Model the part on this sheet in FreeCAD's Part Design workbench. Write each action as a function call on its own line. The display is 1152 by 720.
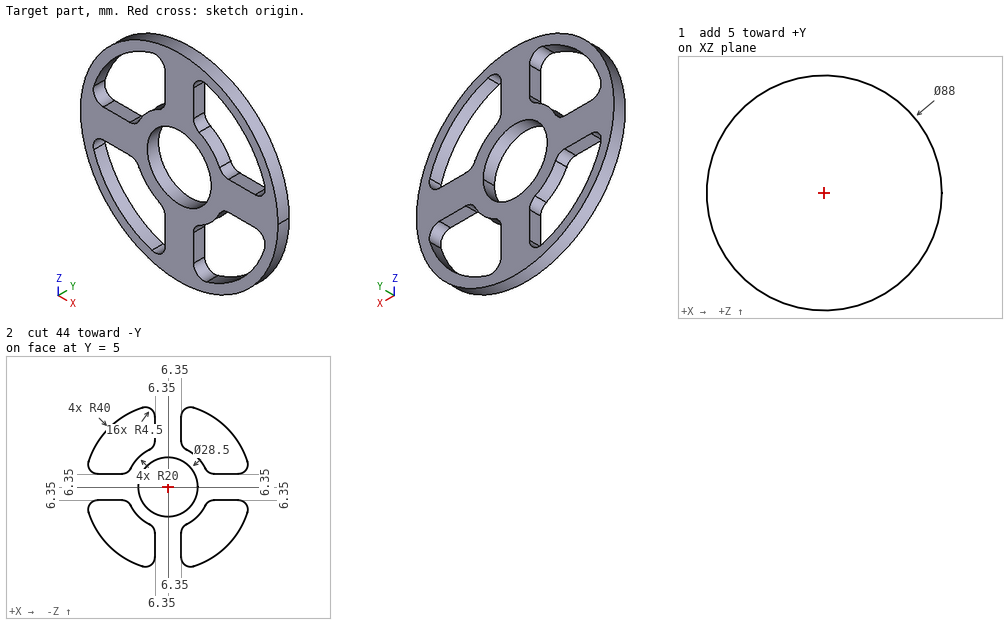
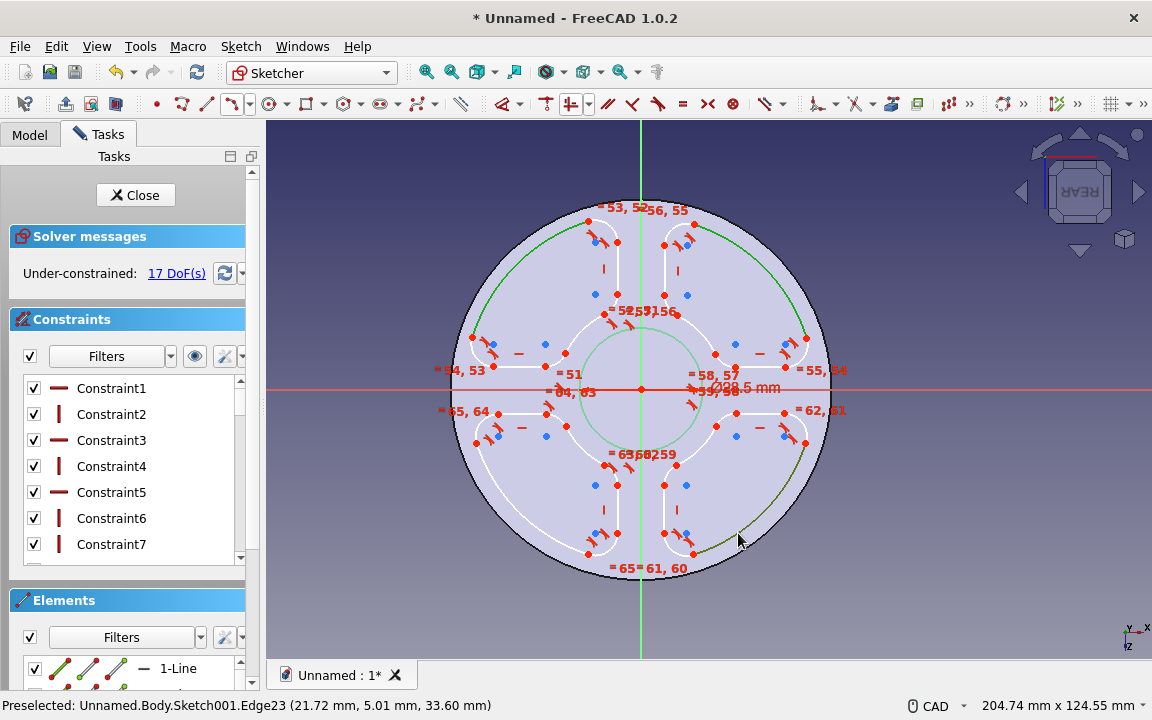
click(499, 488)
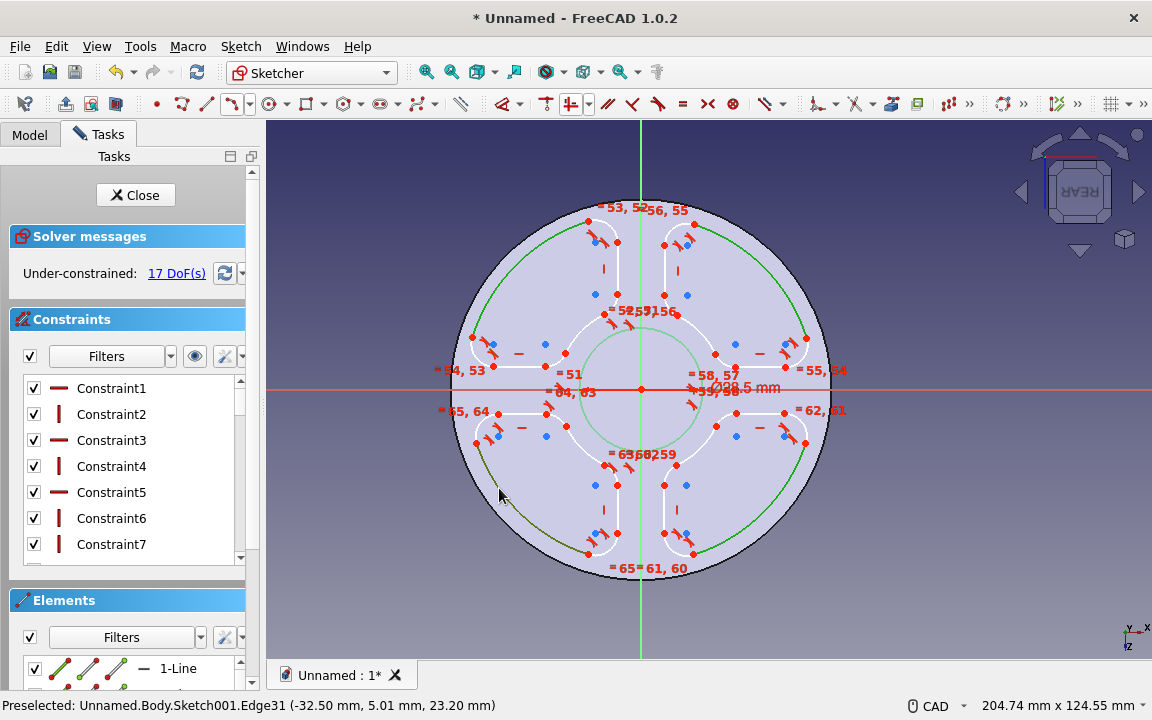
key(e)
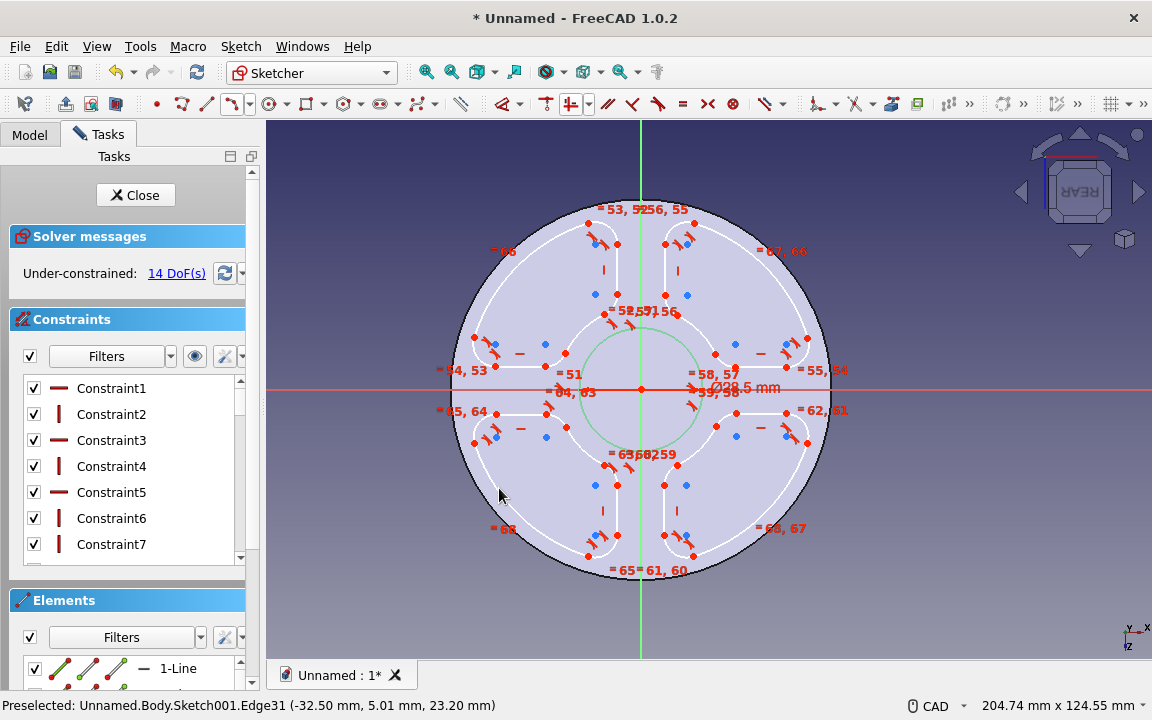
click(590, 323)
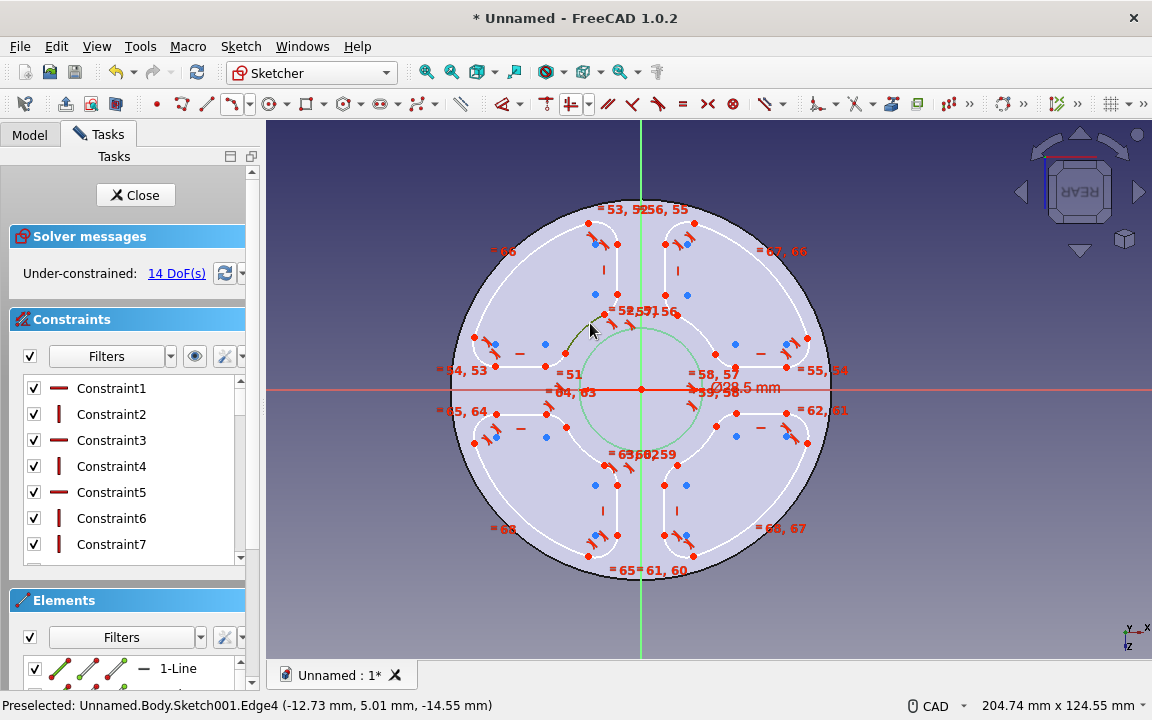
click(707, 340)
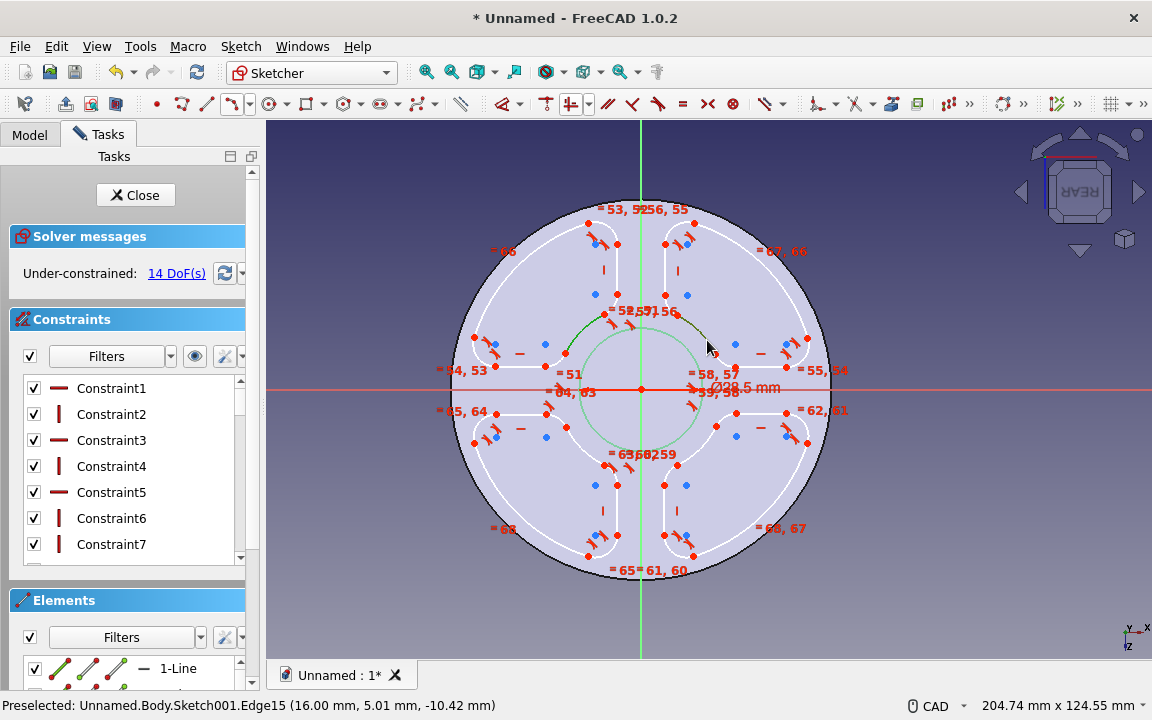
click(691, 457)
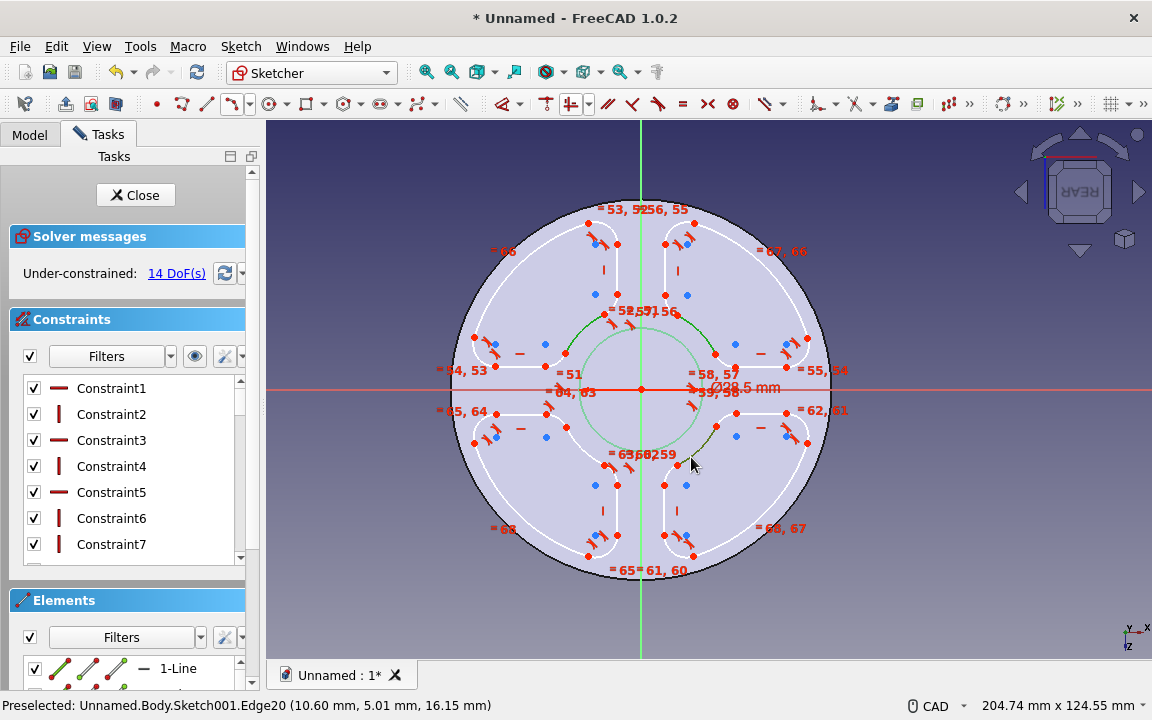
click(575, 441)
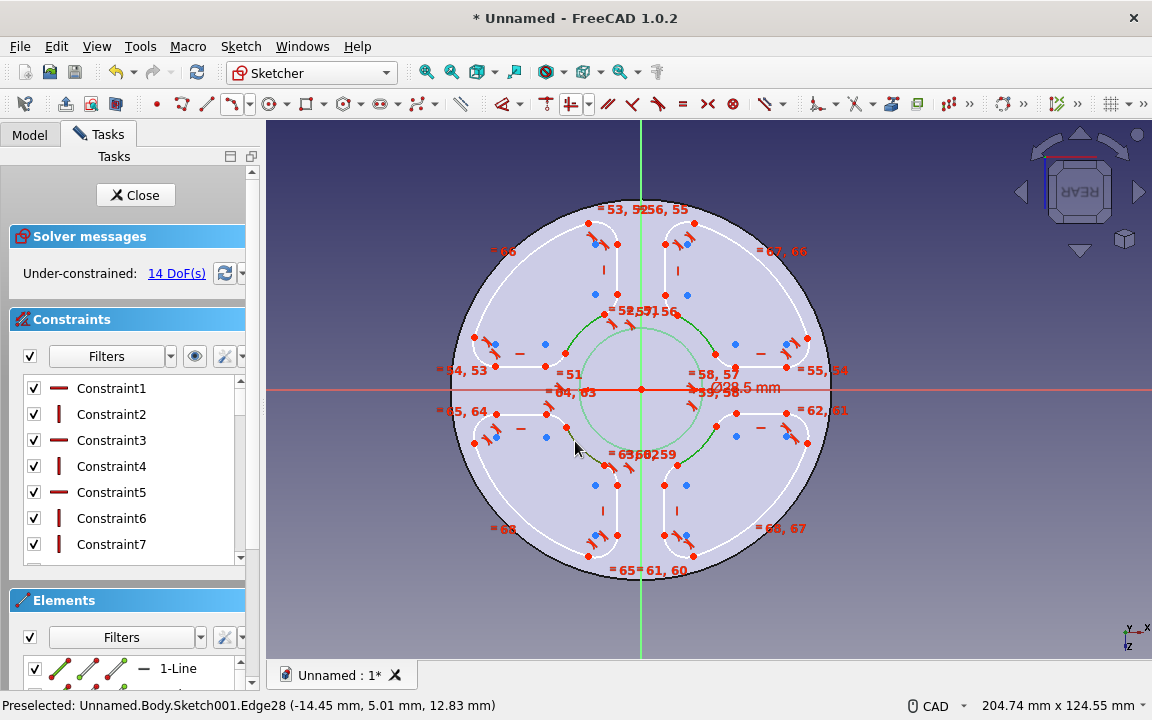
click(683, 104)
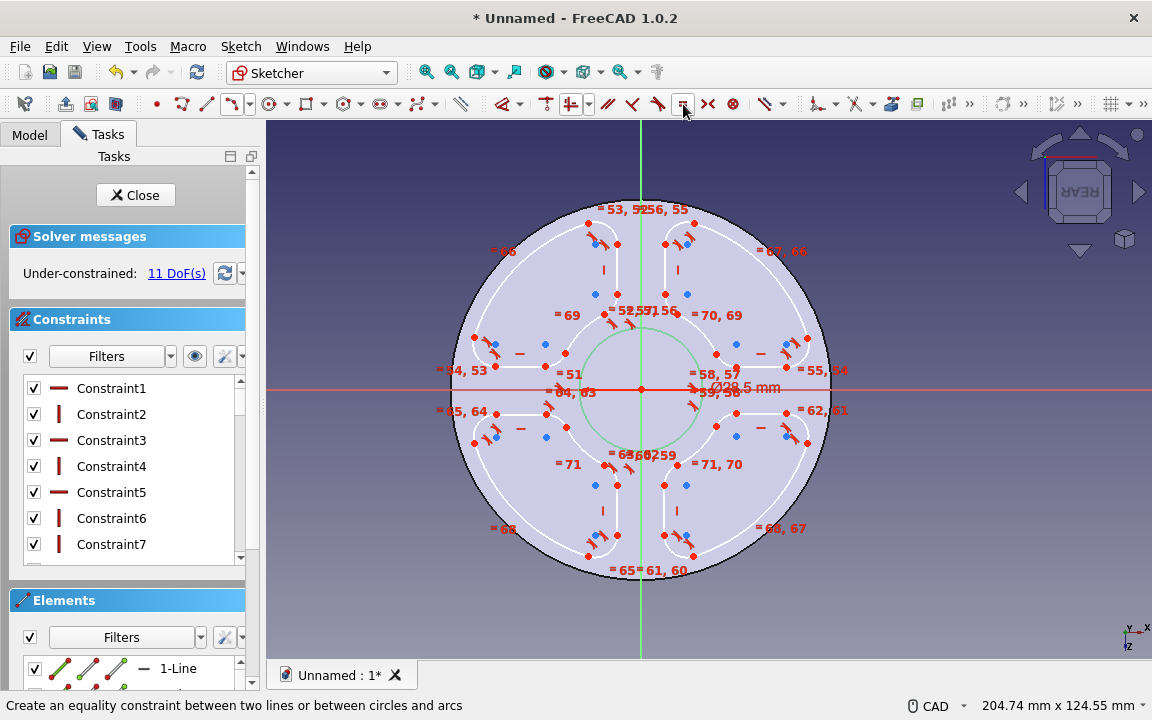
key(d)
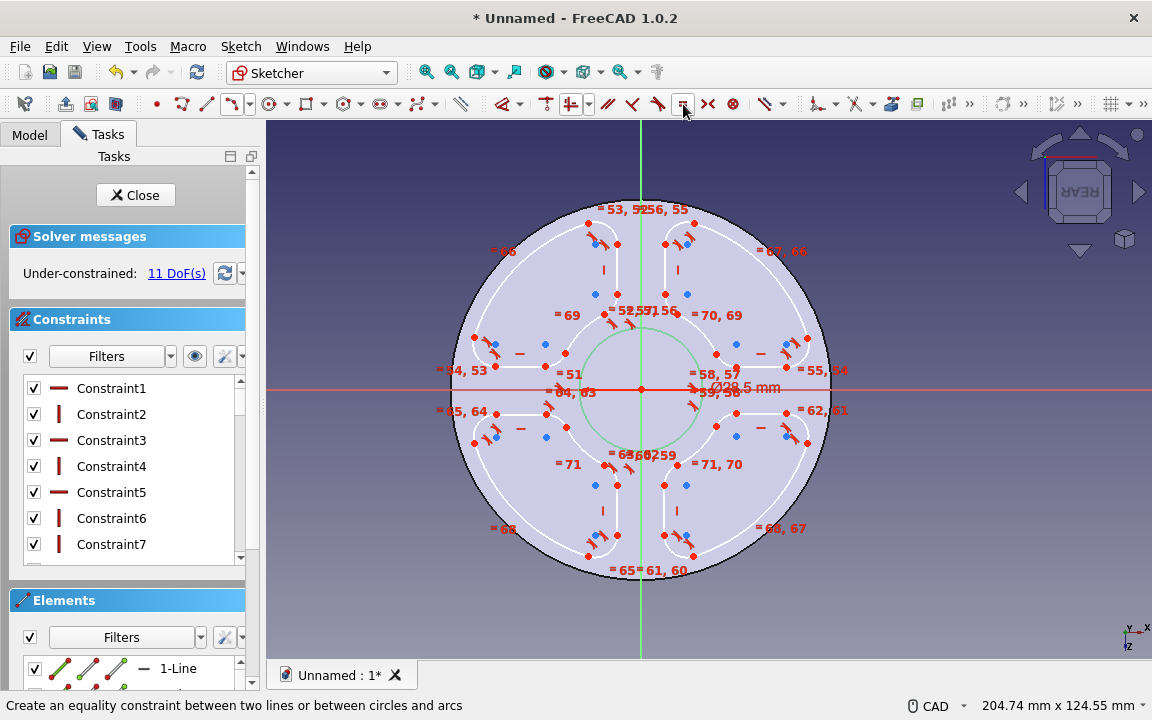
scroll(557, 363, up, 4)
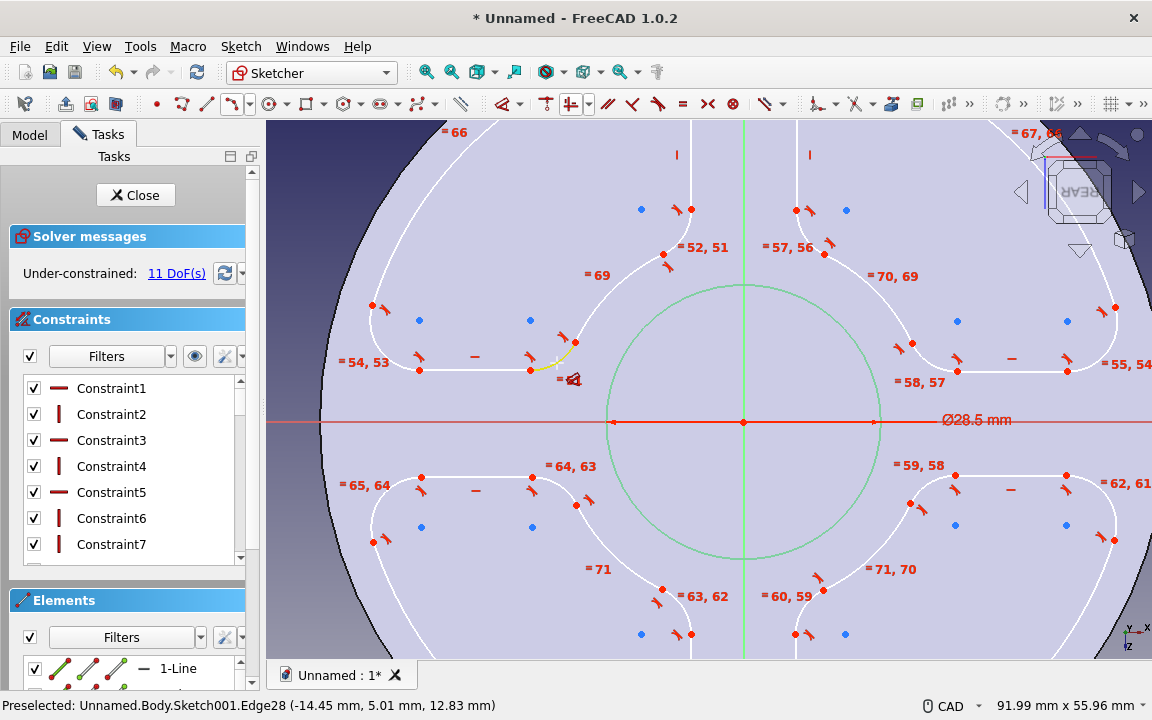
click(557, 363)
click(574, 390)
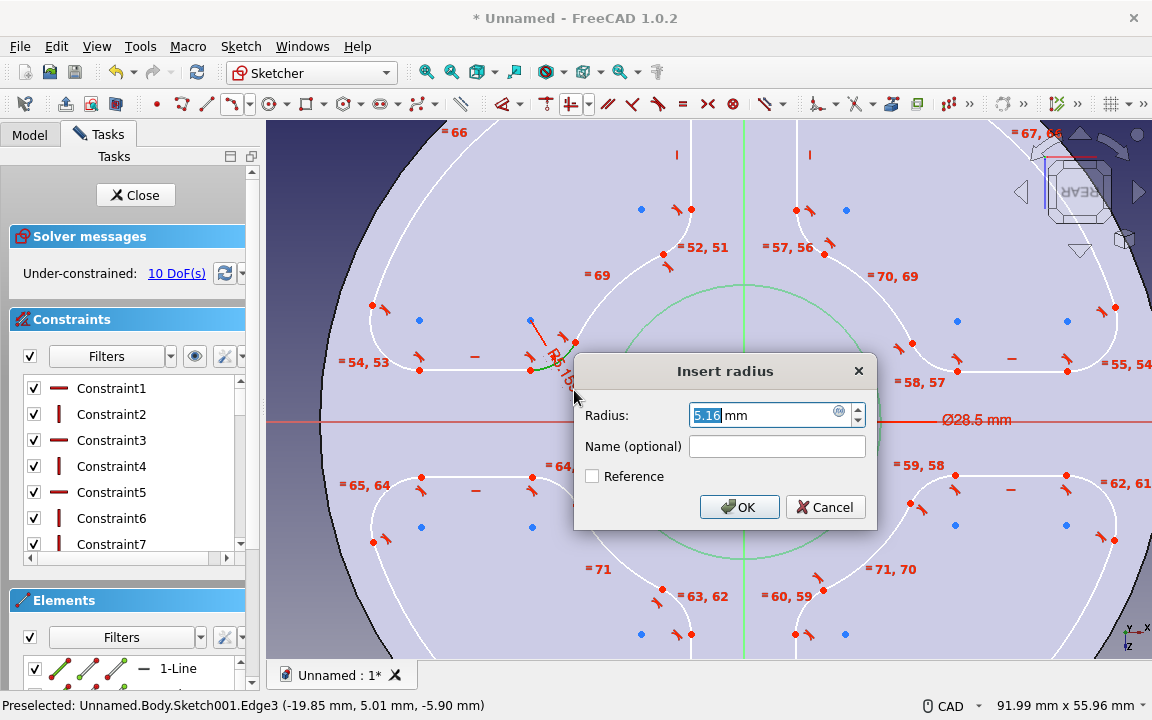
text(4.5)
key(Return)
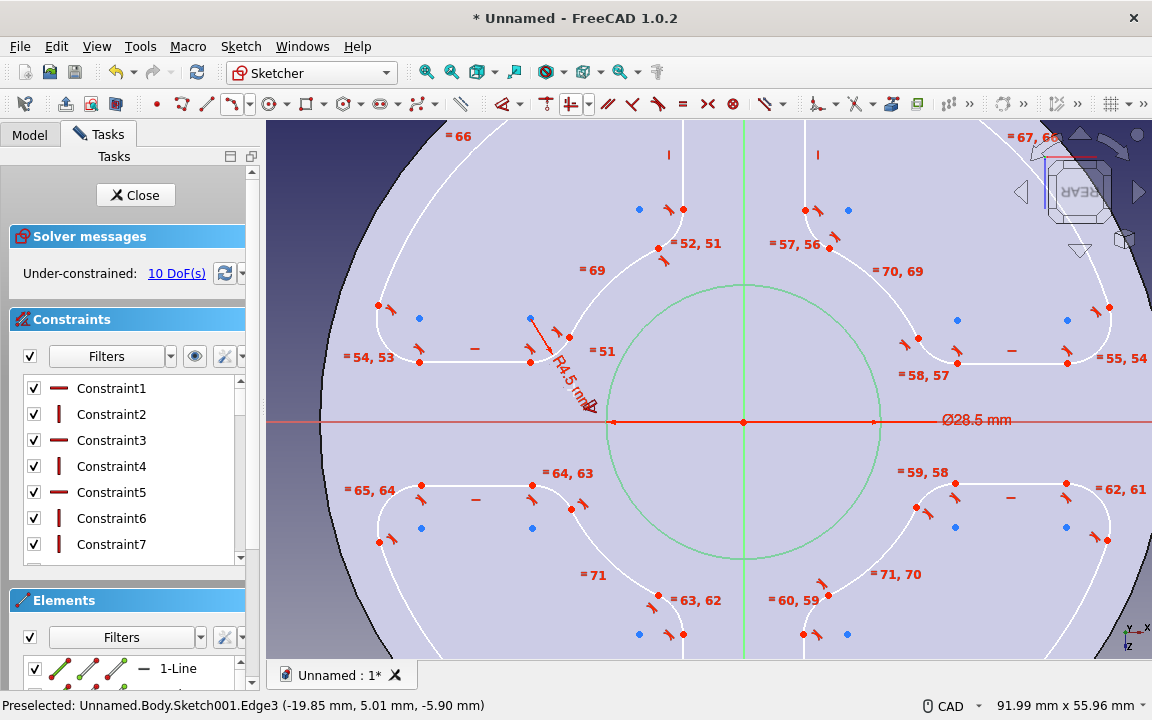
click(626, 269)
click(607, 244)